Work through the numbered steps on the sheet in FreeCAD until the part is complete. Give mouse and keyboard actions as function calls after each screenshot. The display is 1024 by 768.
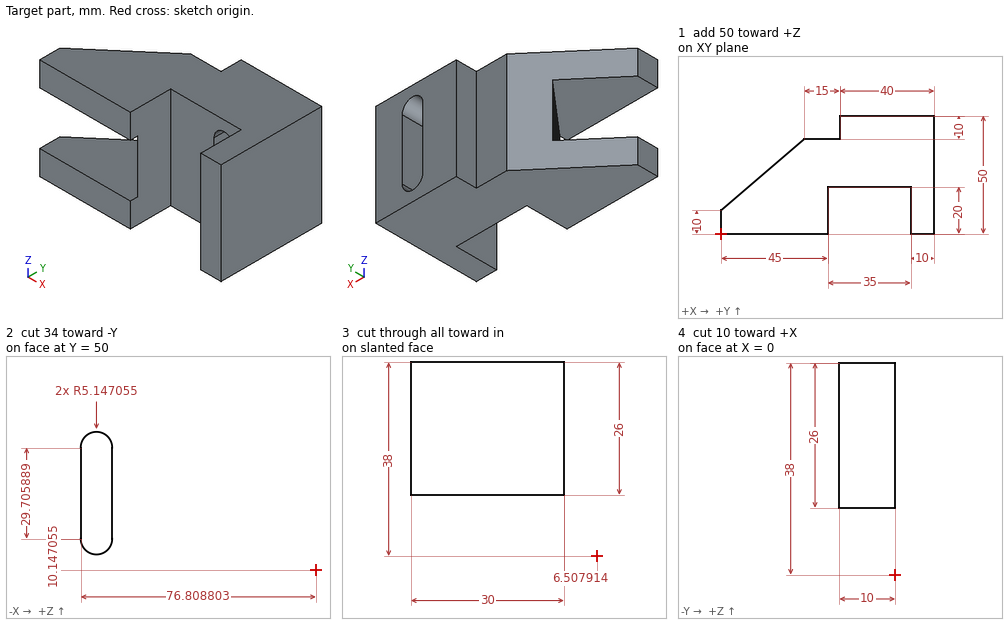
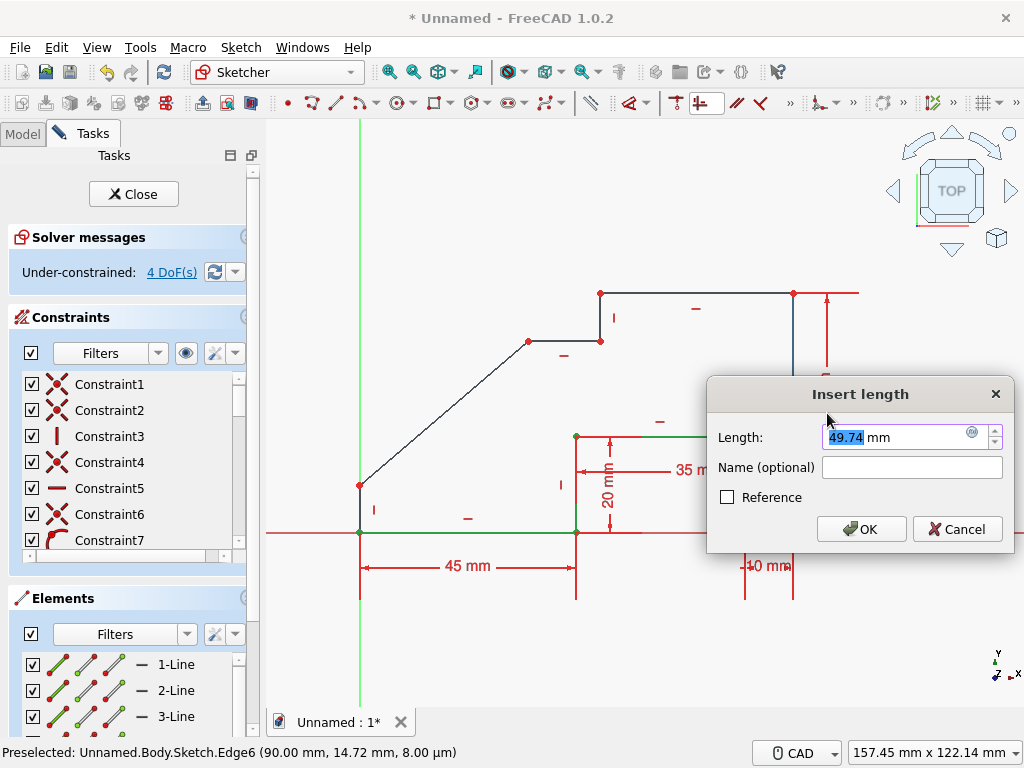
text(50)
key(Return)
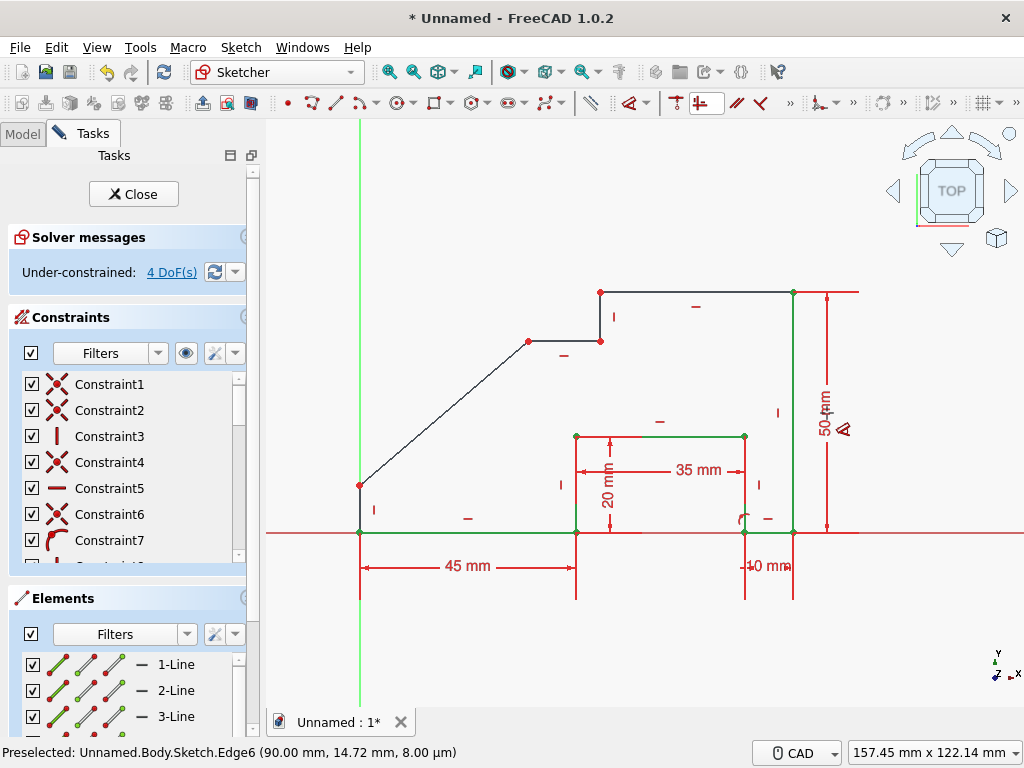
click(735, 292)
click(697, 258)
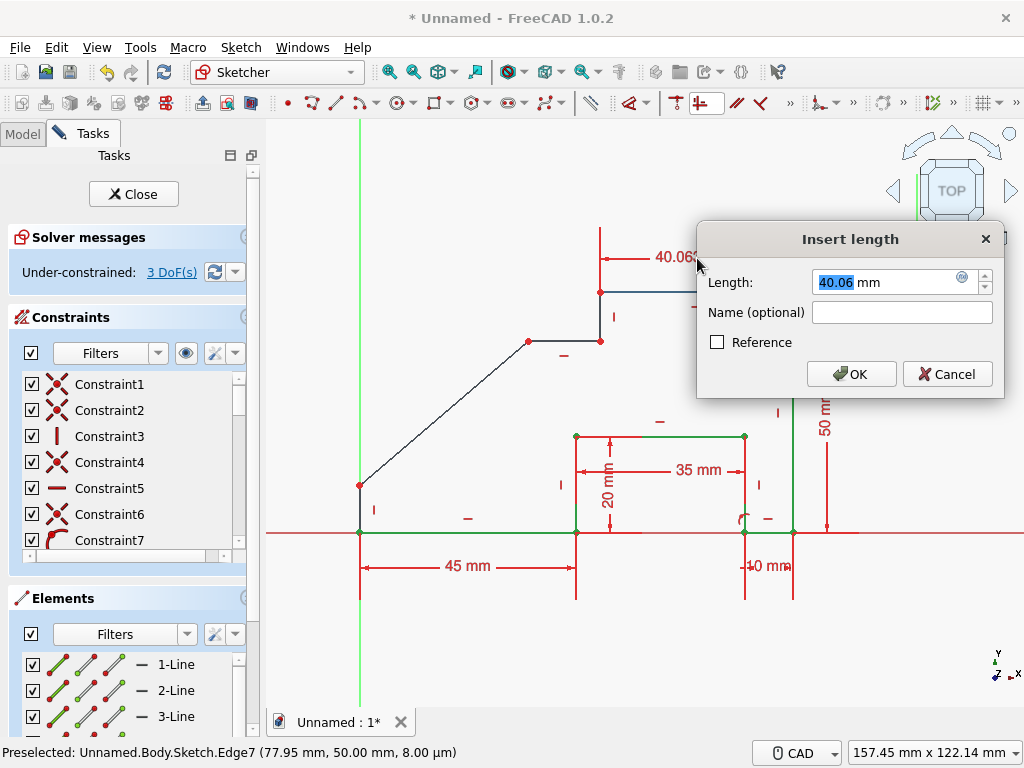
text(40)
key(Return)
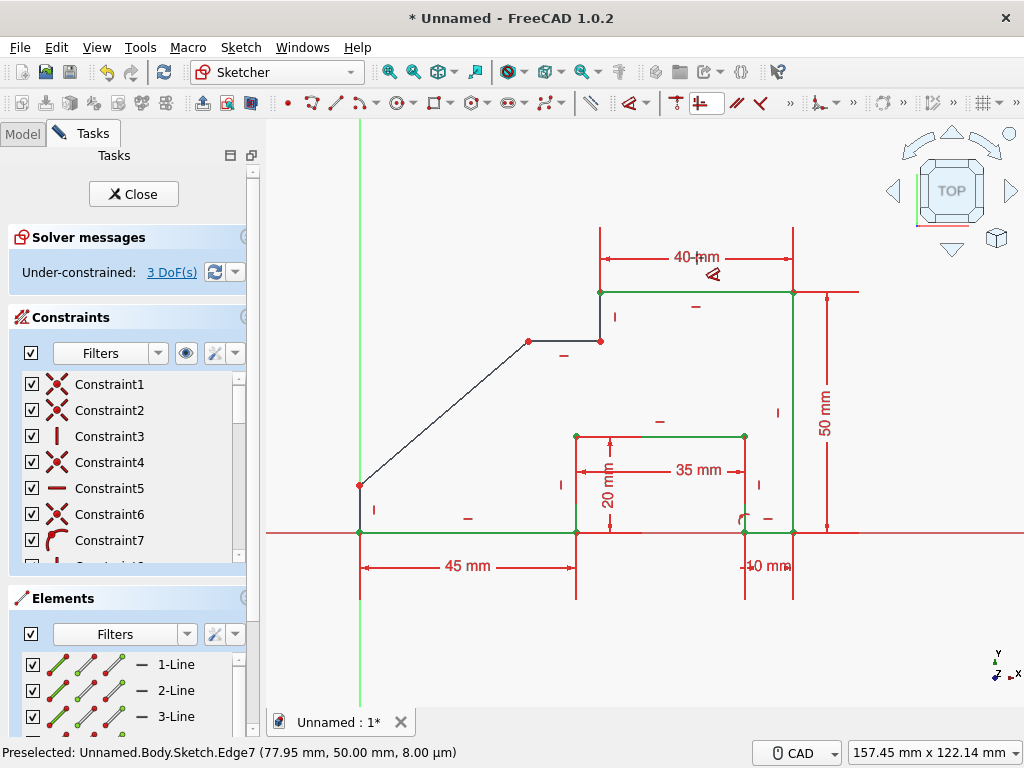
click(600, 307)
click(634, 317)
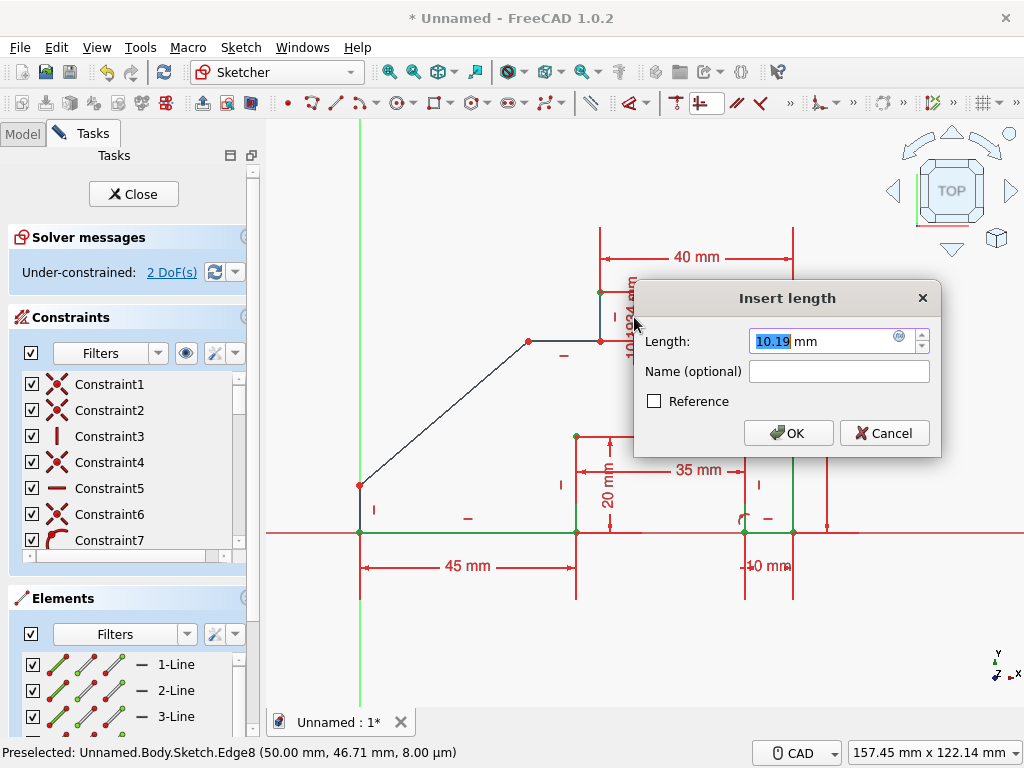
text(10)
key(Return)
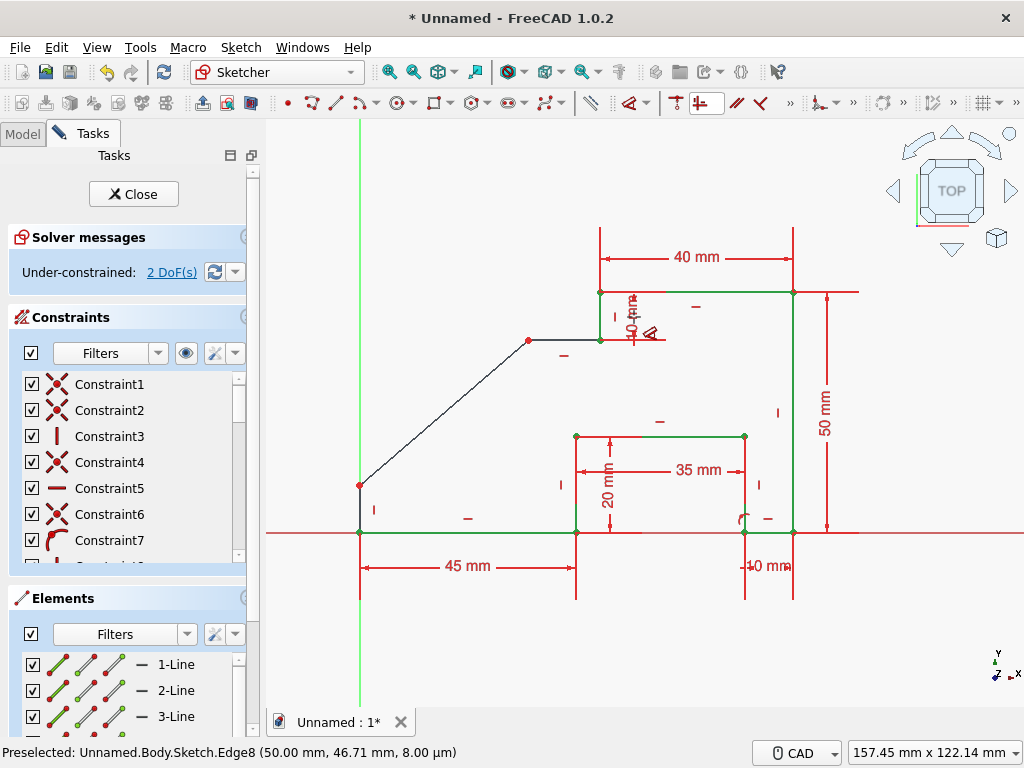
click(579, 340)
click(564, 306)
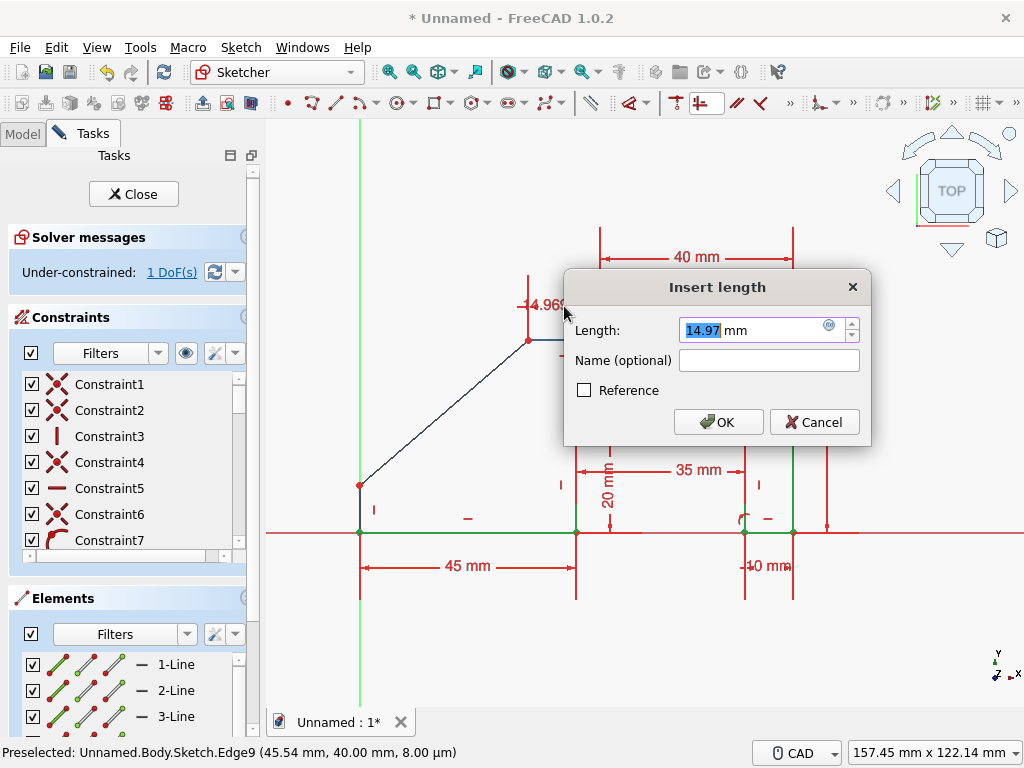
text(15)
key(Return)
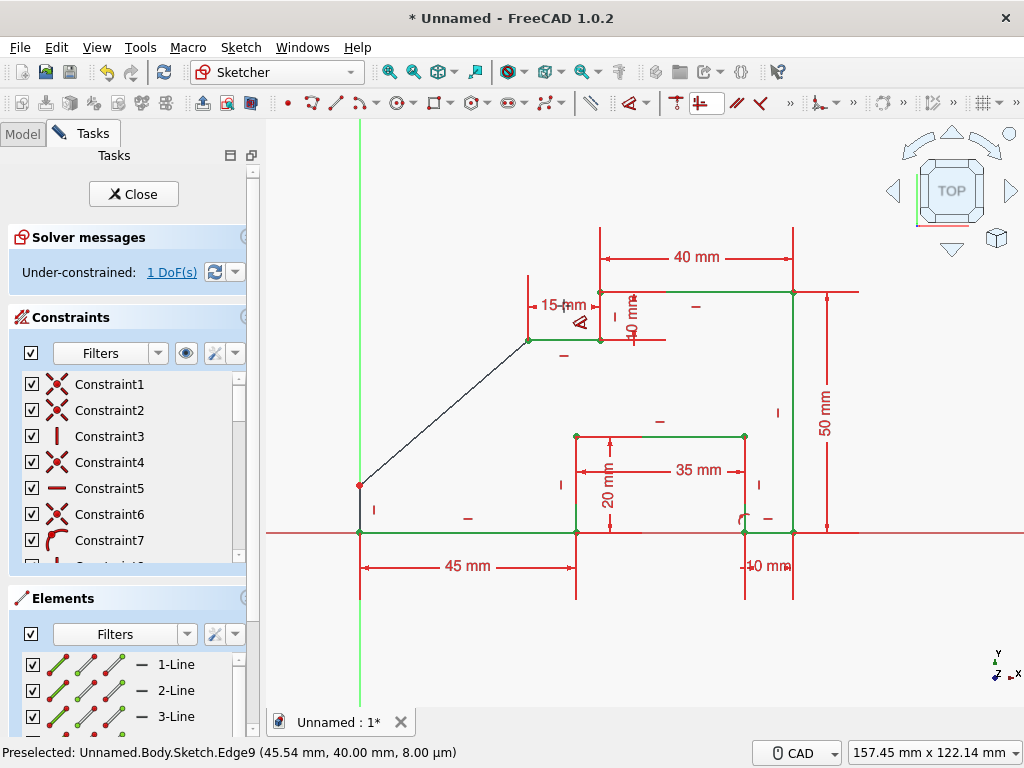
click(360, 500)
click(326, 509)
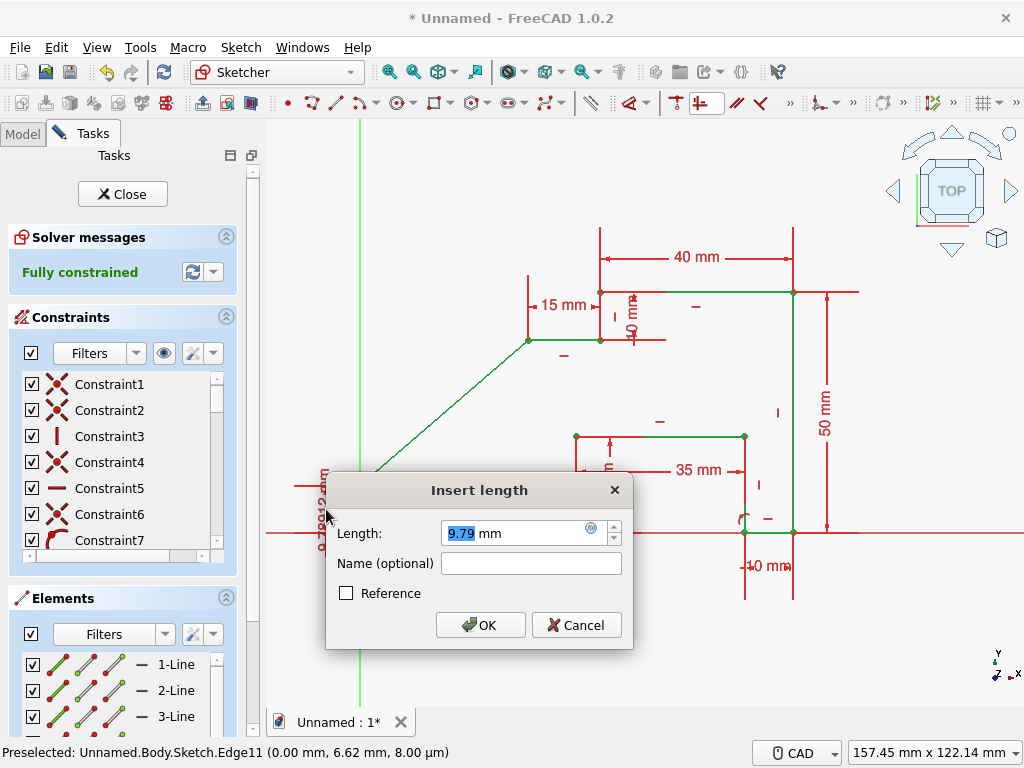
text(10)
key(Return)
key(Escape)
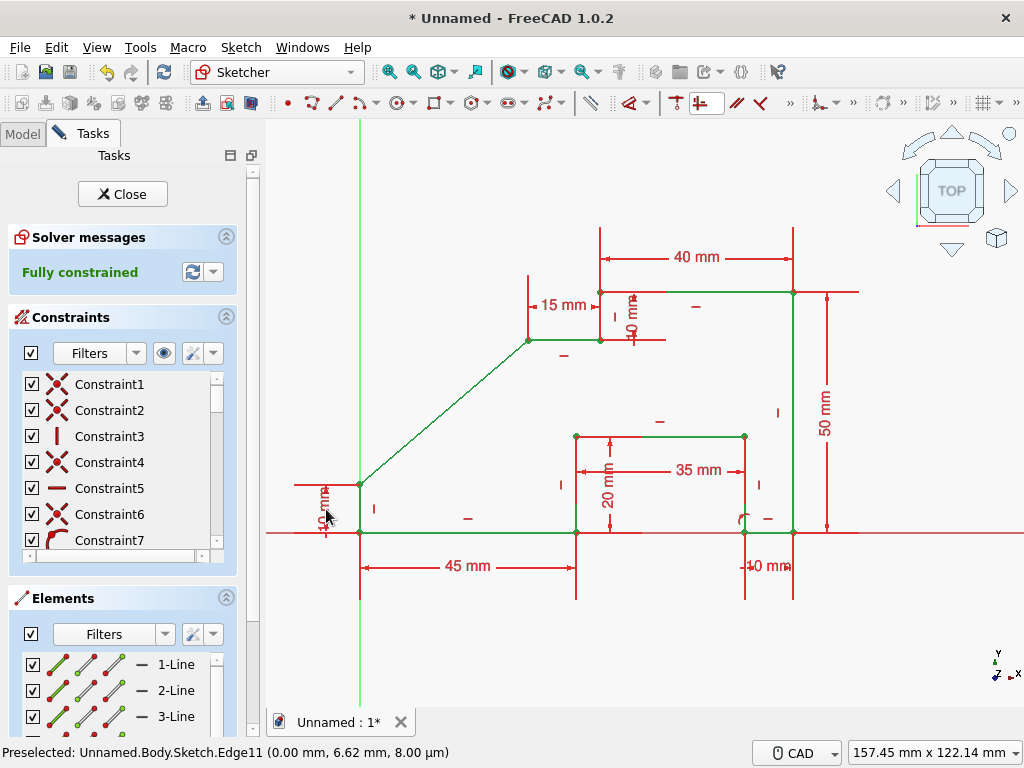
click(123, 194)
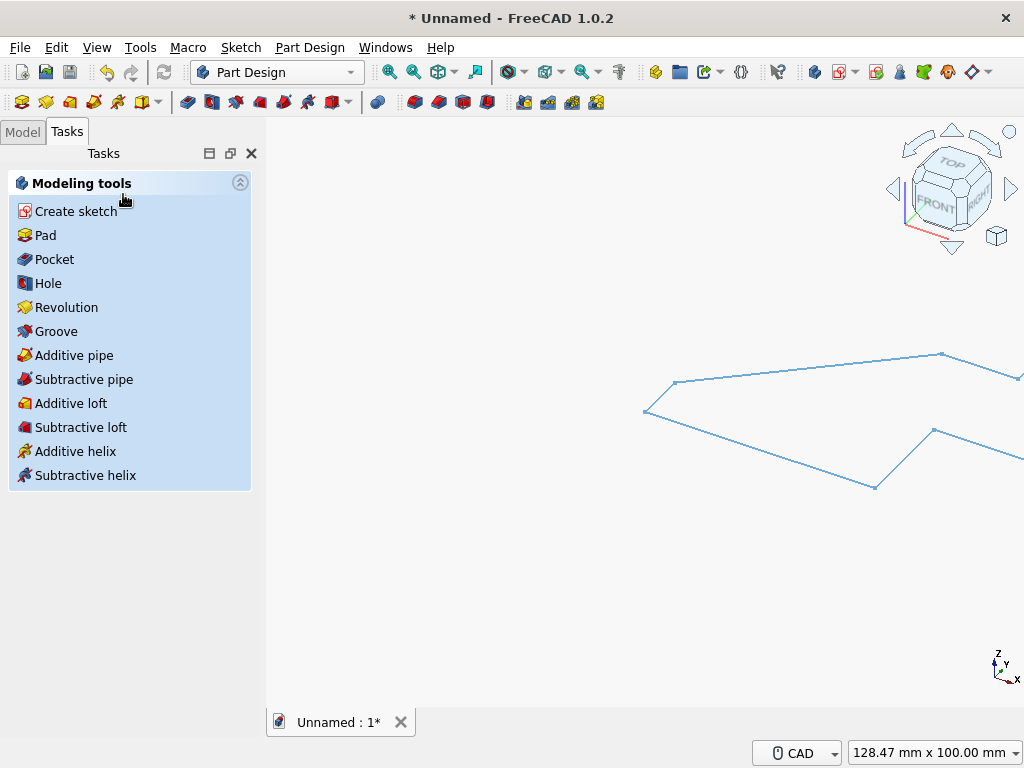
click(22, 102)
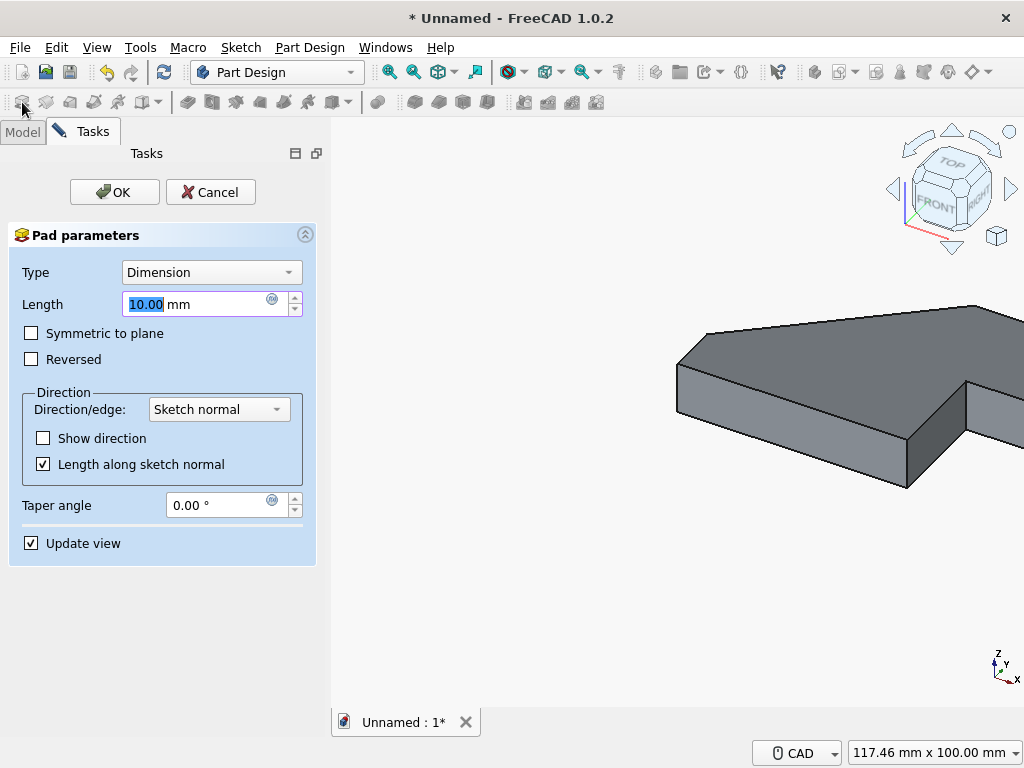
text(50)
key(Tab)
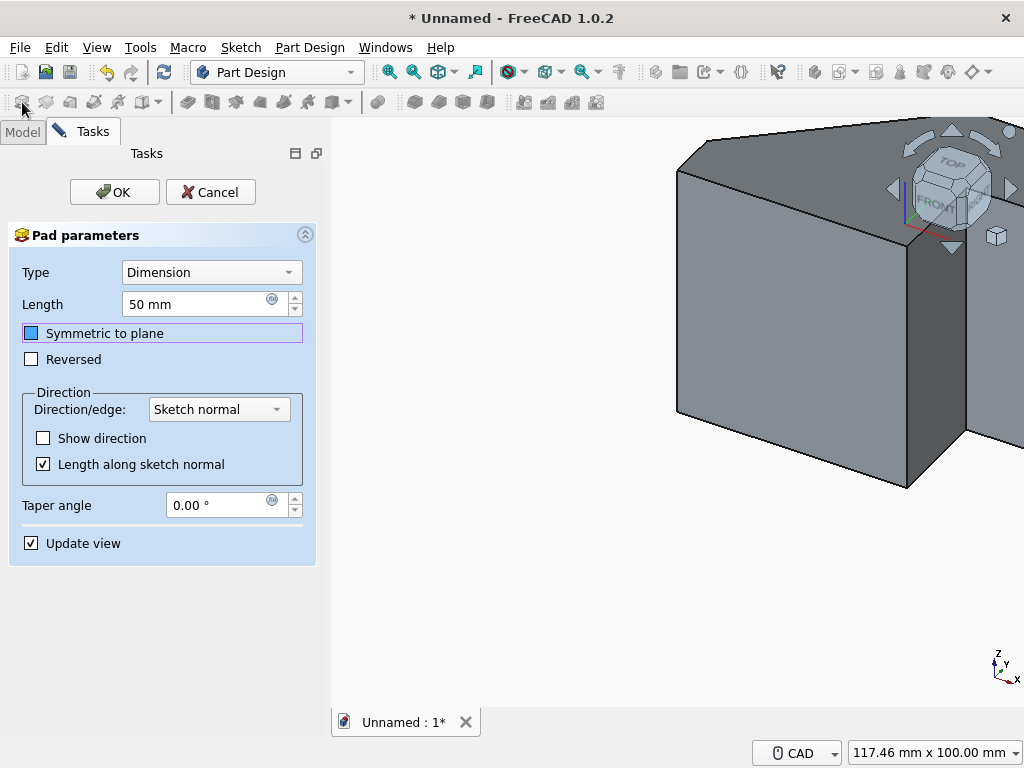
click(115, 192)